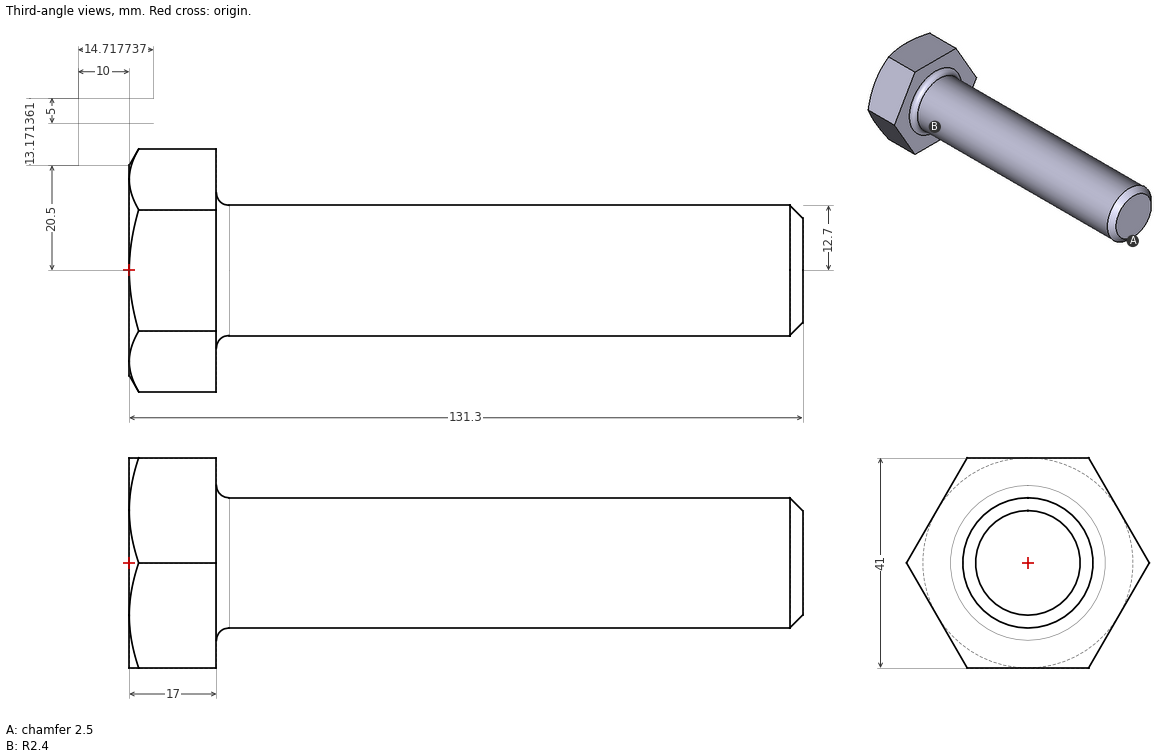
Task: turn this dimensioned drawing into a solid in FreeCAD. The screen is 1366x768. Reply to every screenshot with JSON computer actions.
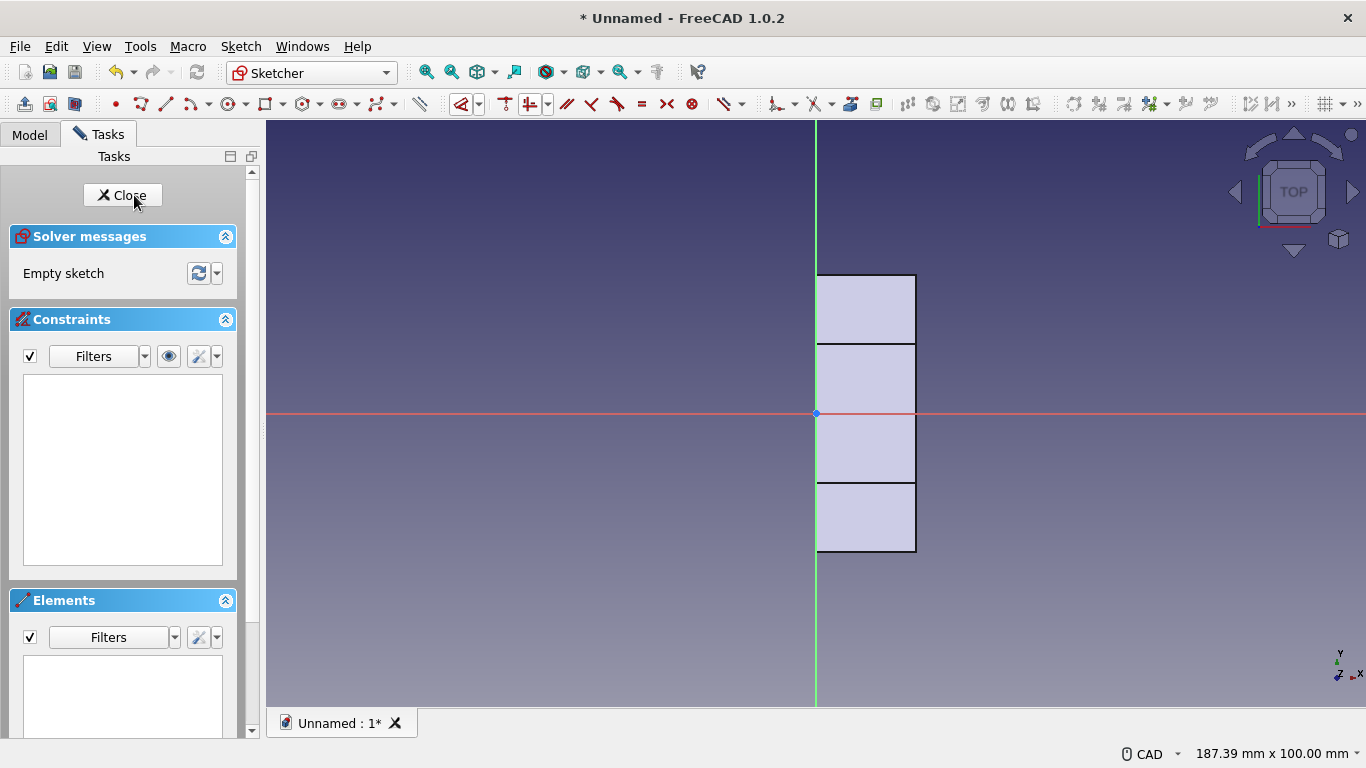
{"action": "scroll", "coordinate": [294, 489], "scroll_direction": "down", "scroll_amount": 2}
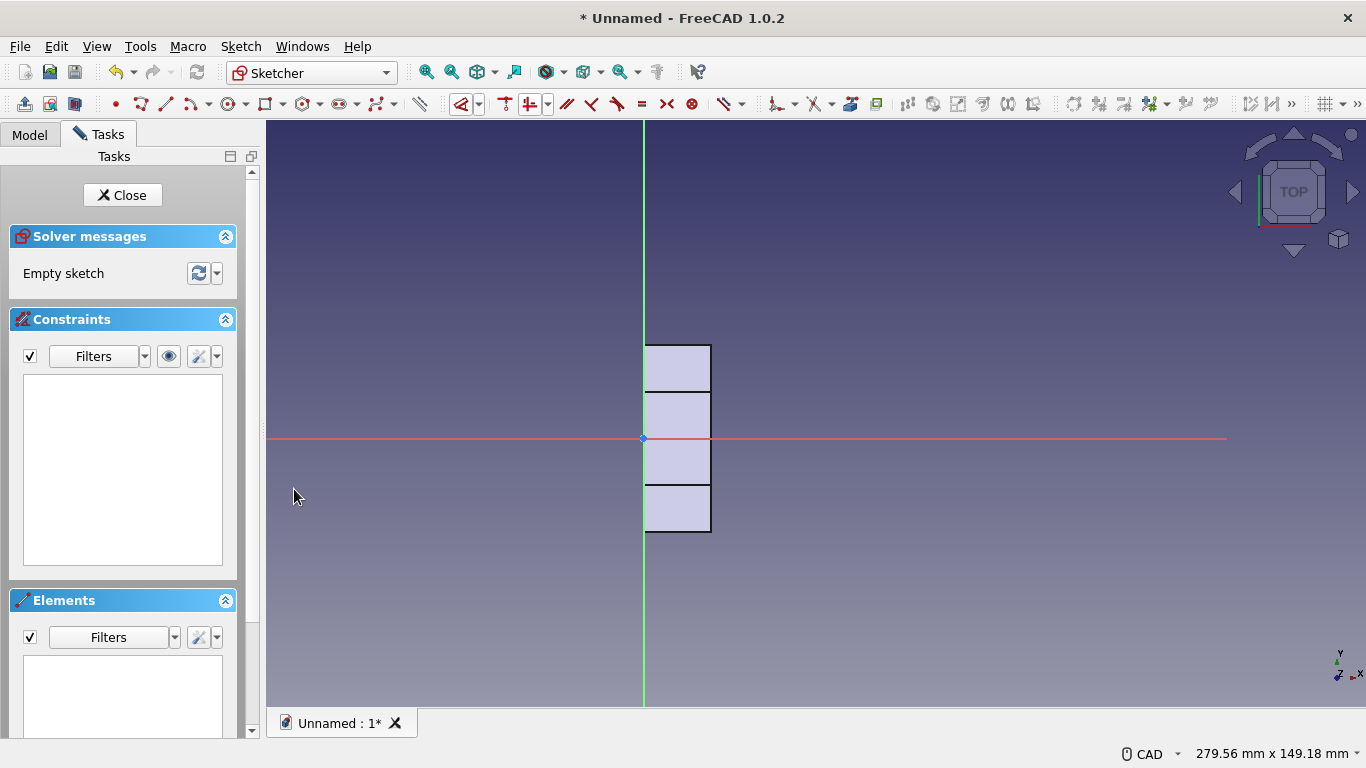
{"action": "key", "text": "g r"}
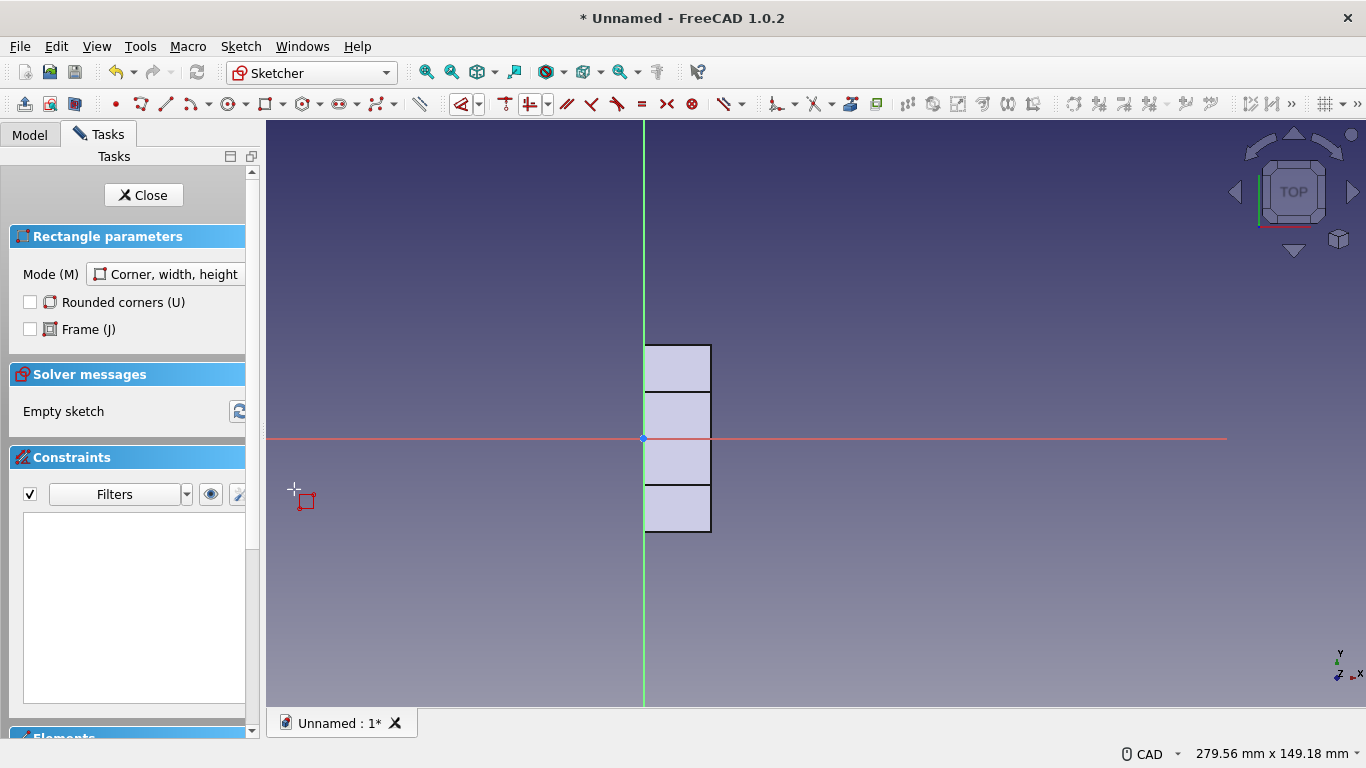
{"action": "left_click", "coordinate": [644, 439]}
{"action": "left_click", "coordinate": [1161, 389]}
{"action": "key", "text": "Escape"}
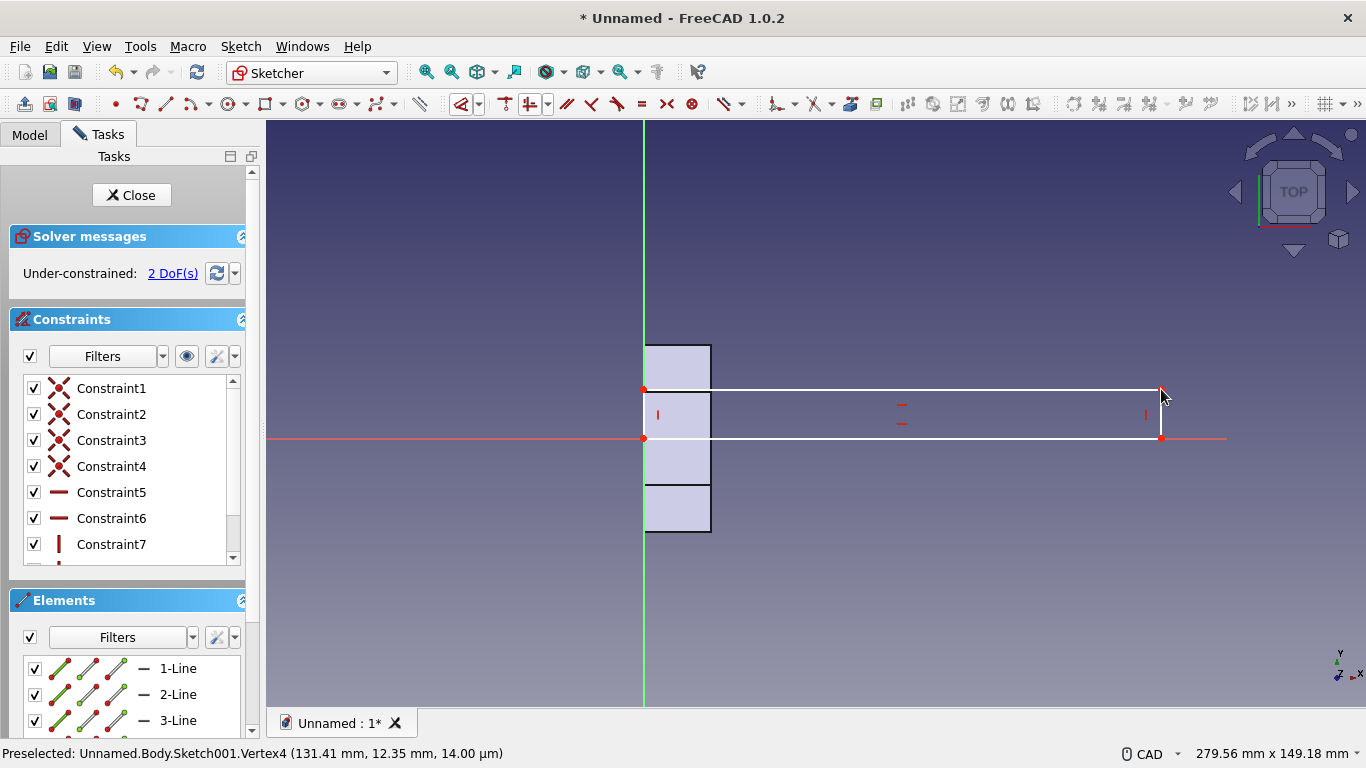
{"action": "key", "text": "d"}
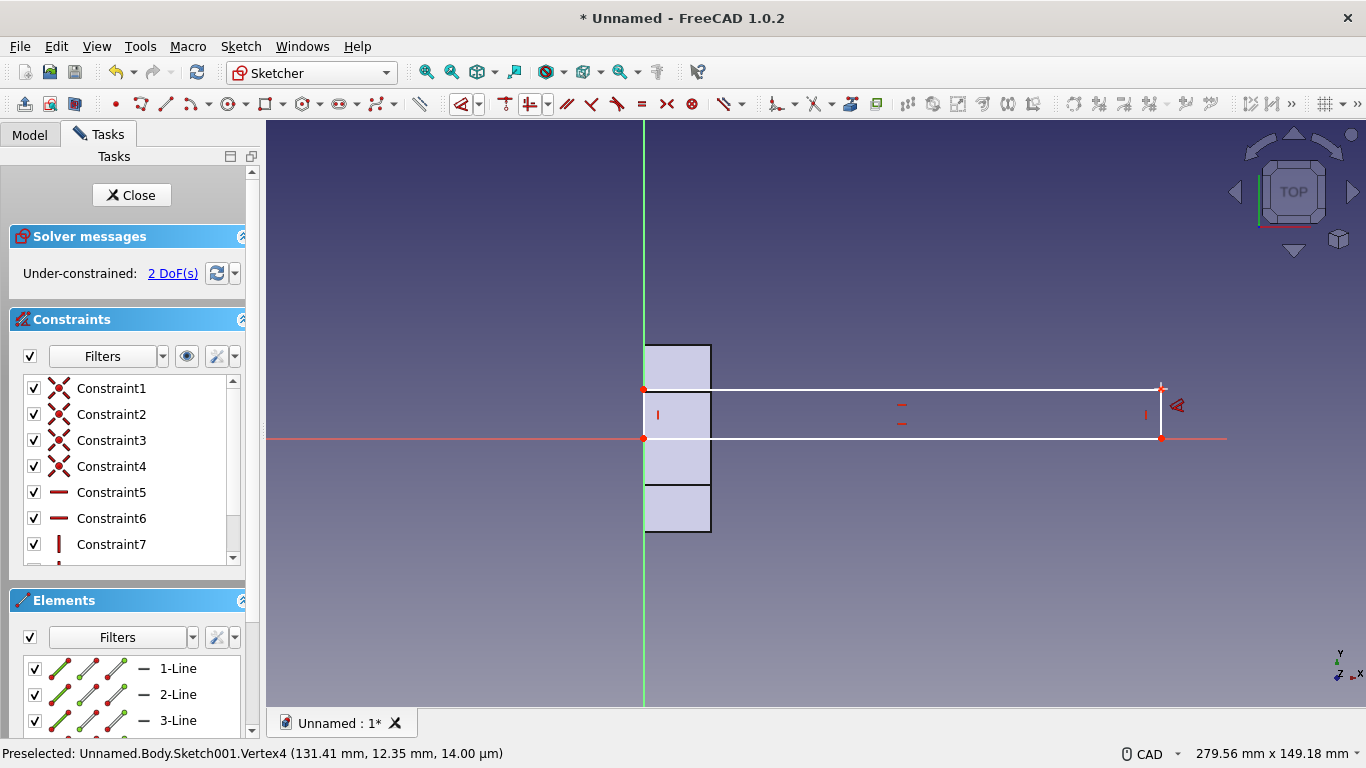
{"action": "left_click", "coordinate": [1161, 424]}
{"action": "left_click", "coordinate": [1195, 414]}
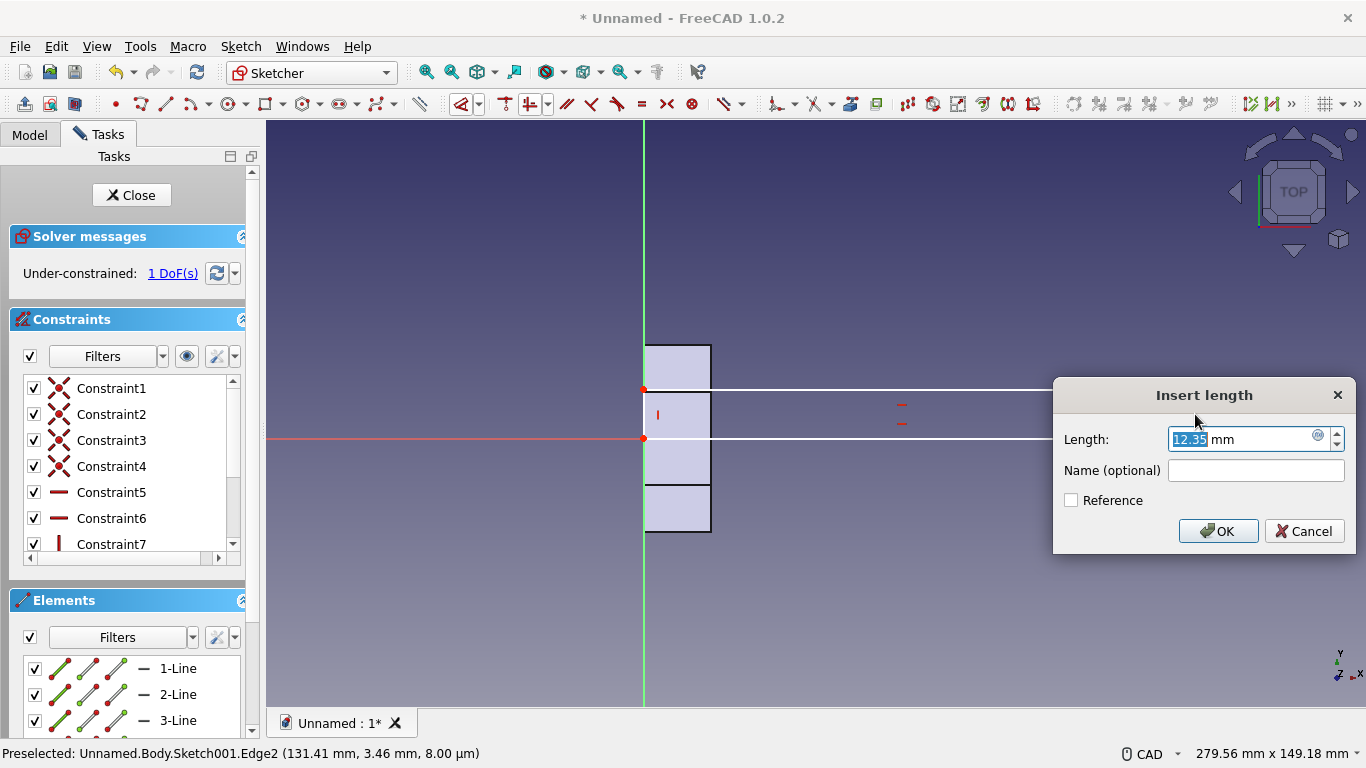
{"action": "type", "text": "12.7"}
{"action": "key", "text": "Return"}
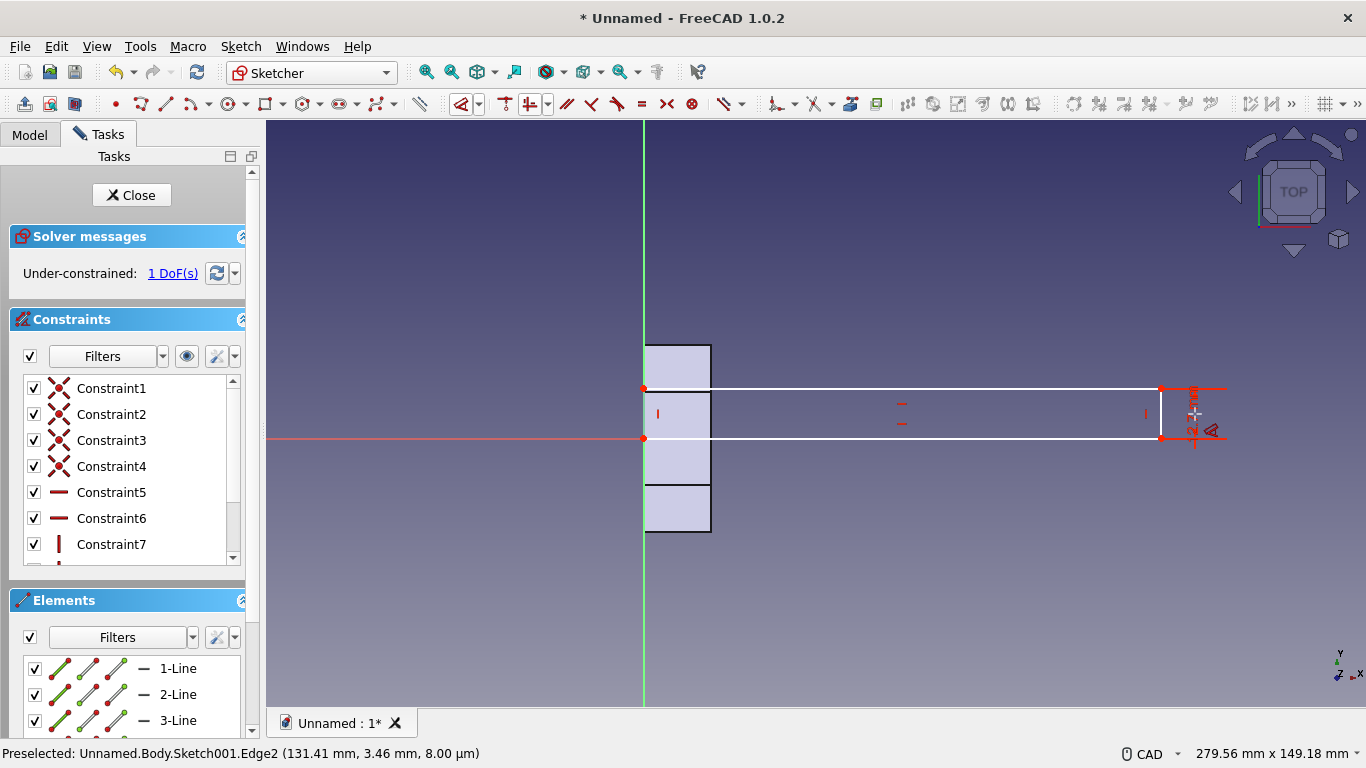
{"action": "left_click", "coordinate": [799, 439]}
{"action": "left_click", "coordinate": [902, 473]}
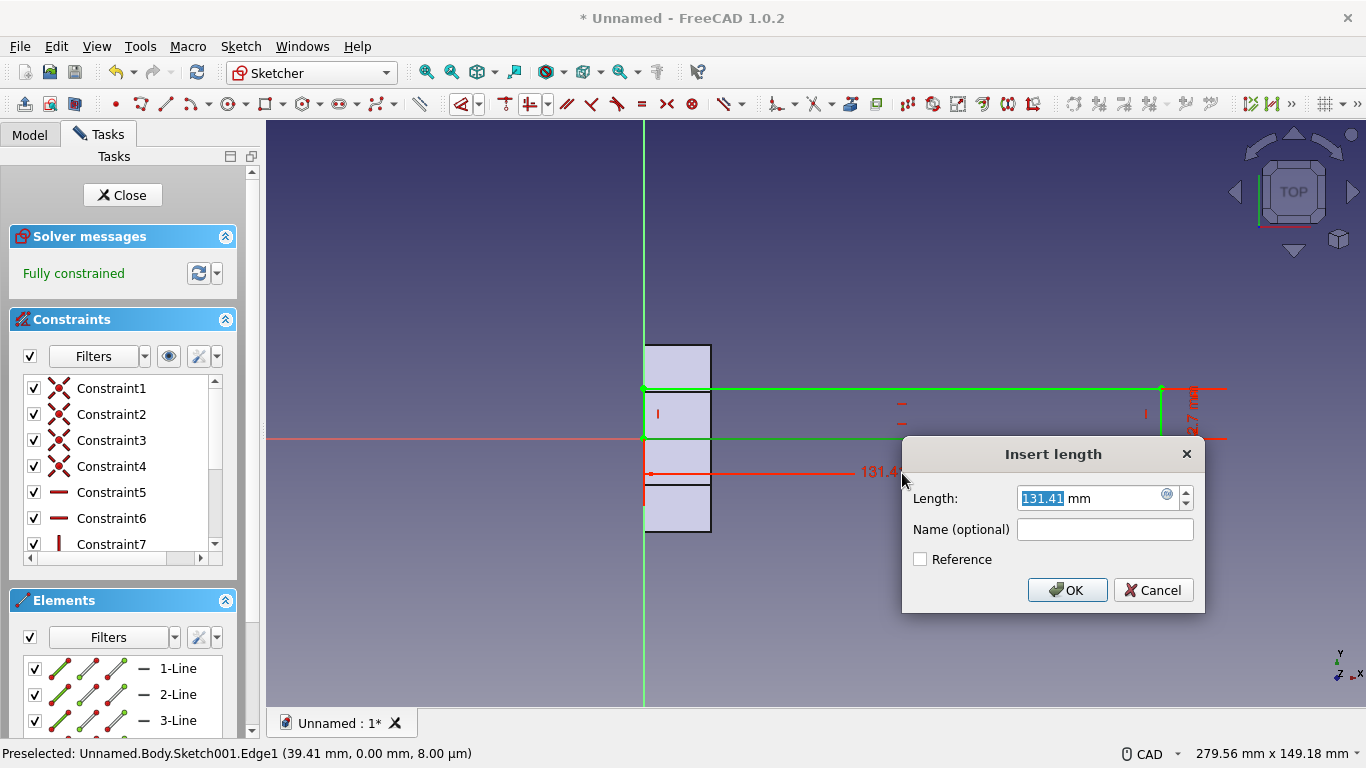
{"action": "type", "text": "131.3"}
{"action": "key", "text": "Return"}
{"action": "key", "text": "Escape"}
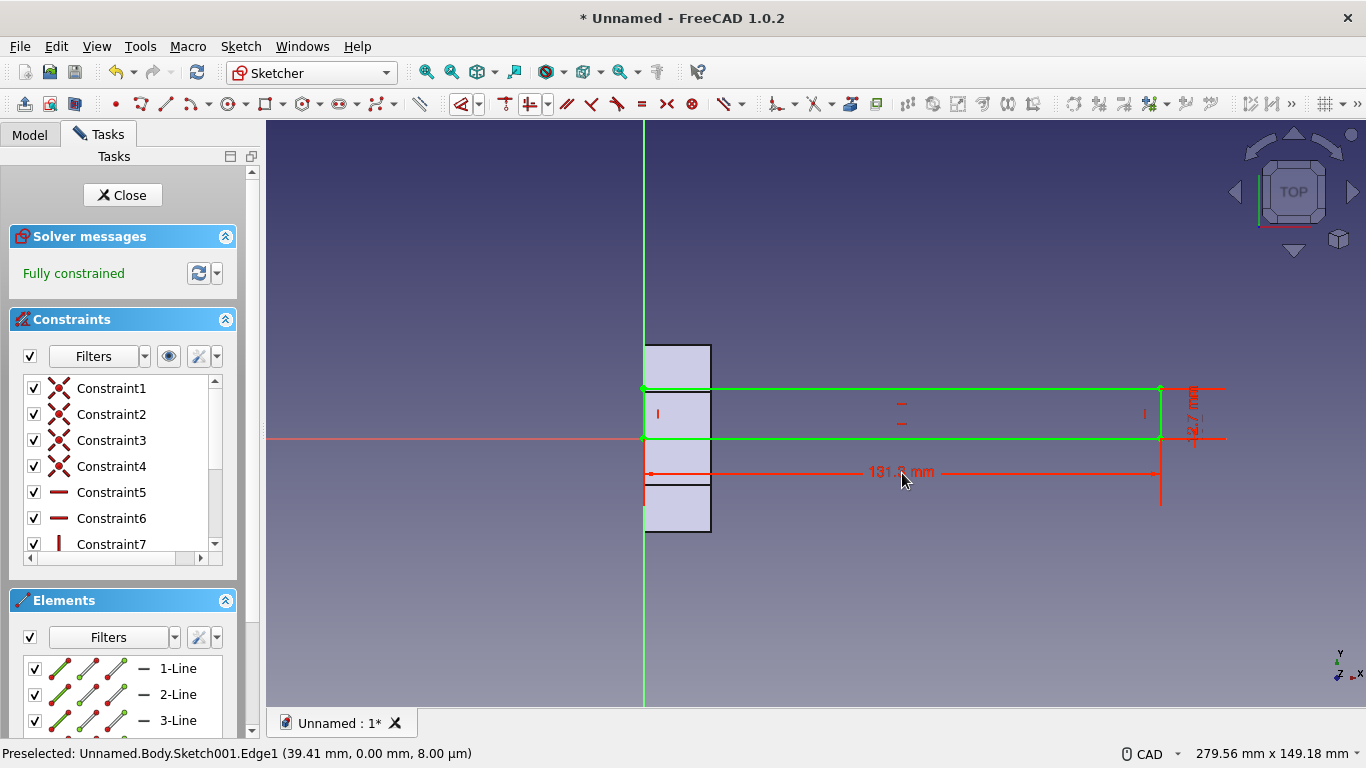
{"action": "left_click", "coordinate": [123, 195]}